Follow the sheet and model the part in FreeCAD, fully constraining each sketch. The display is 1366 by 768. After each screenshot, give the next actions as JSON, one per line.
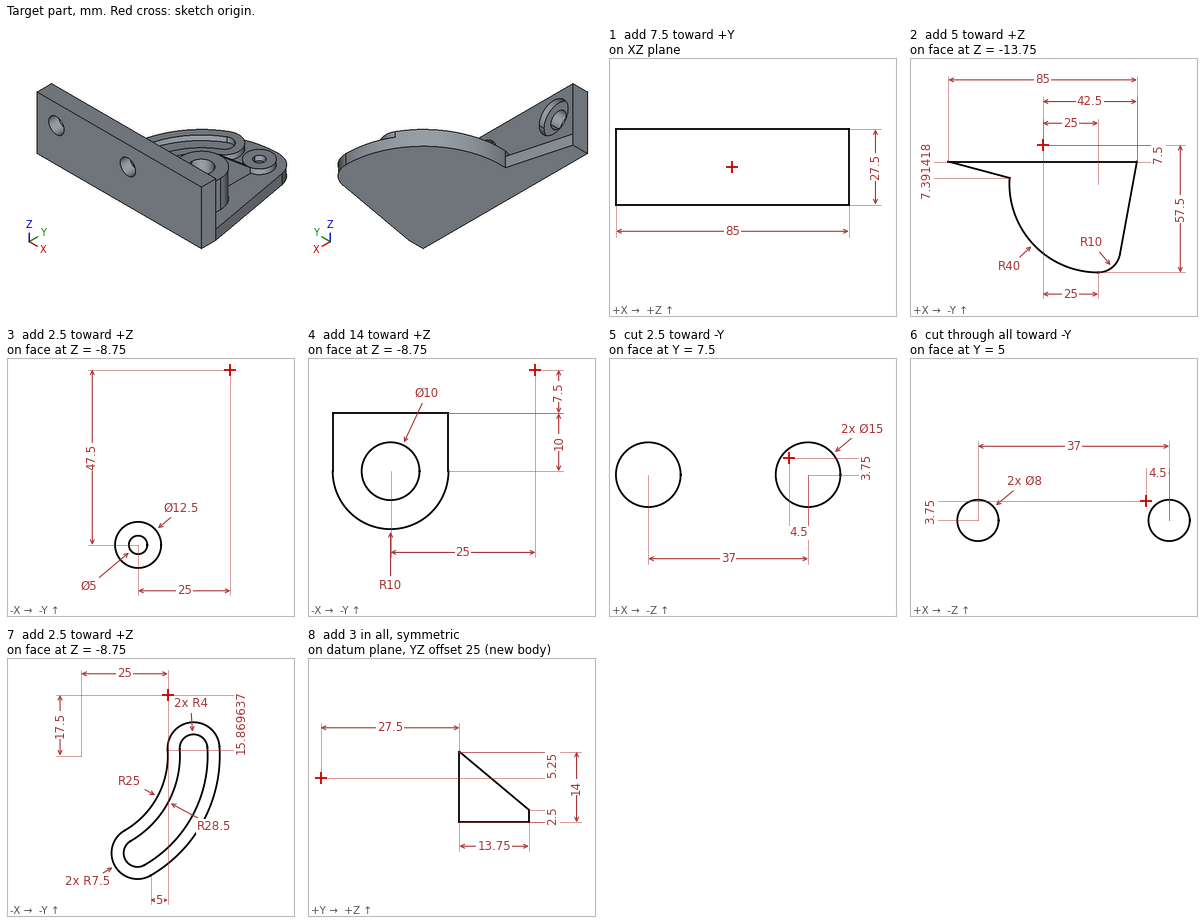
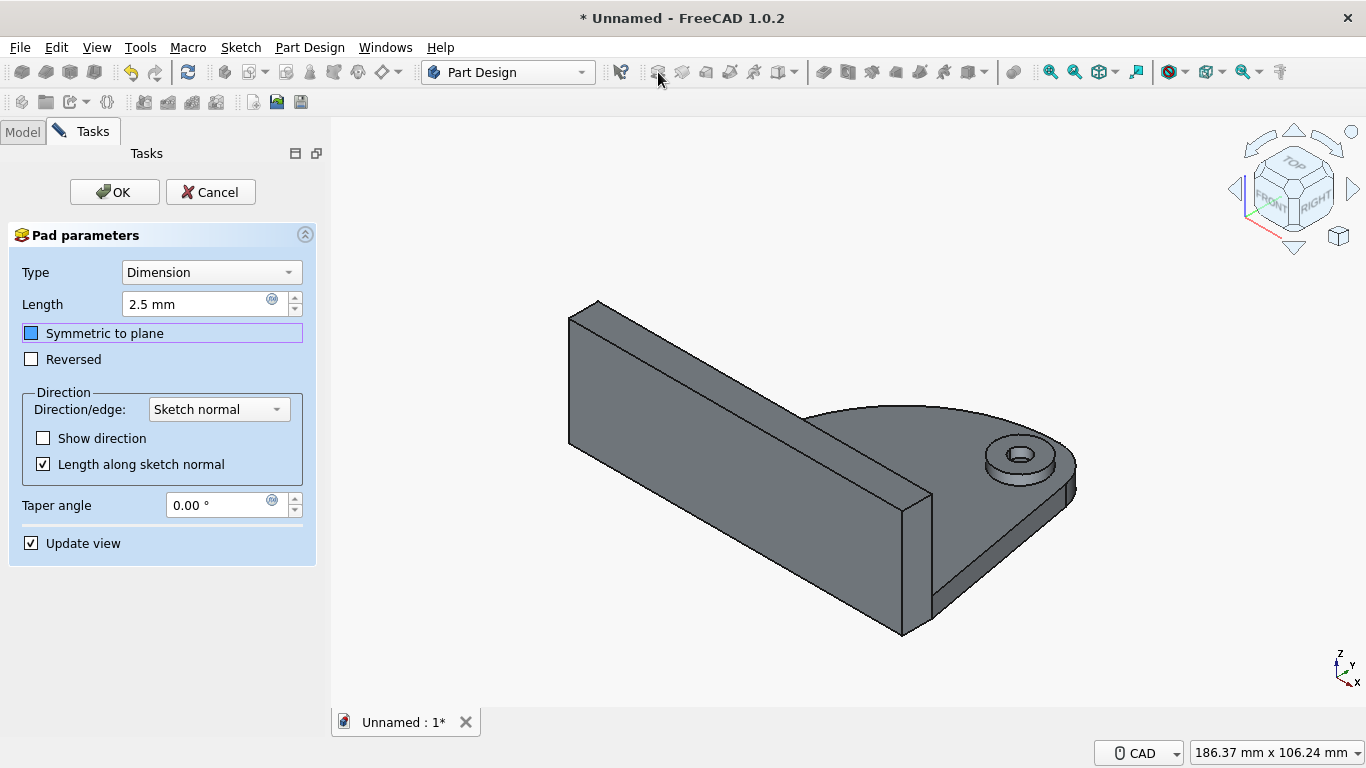
{"action": "left_click", "coordinate": [115, 192]}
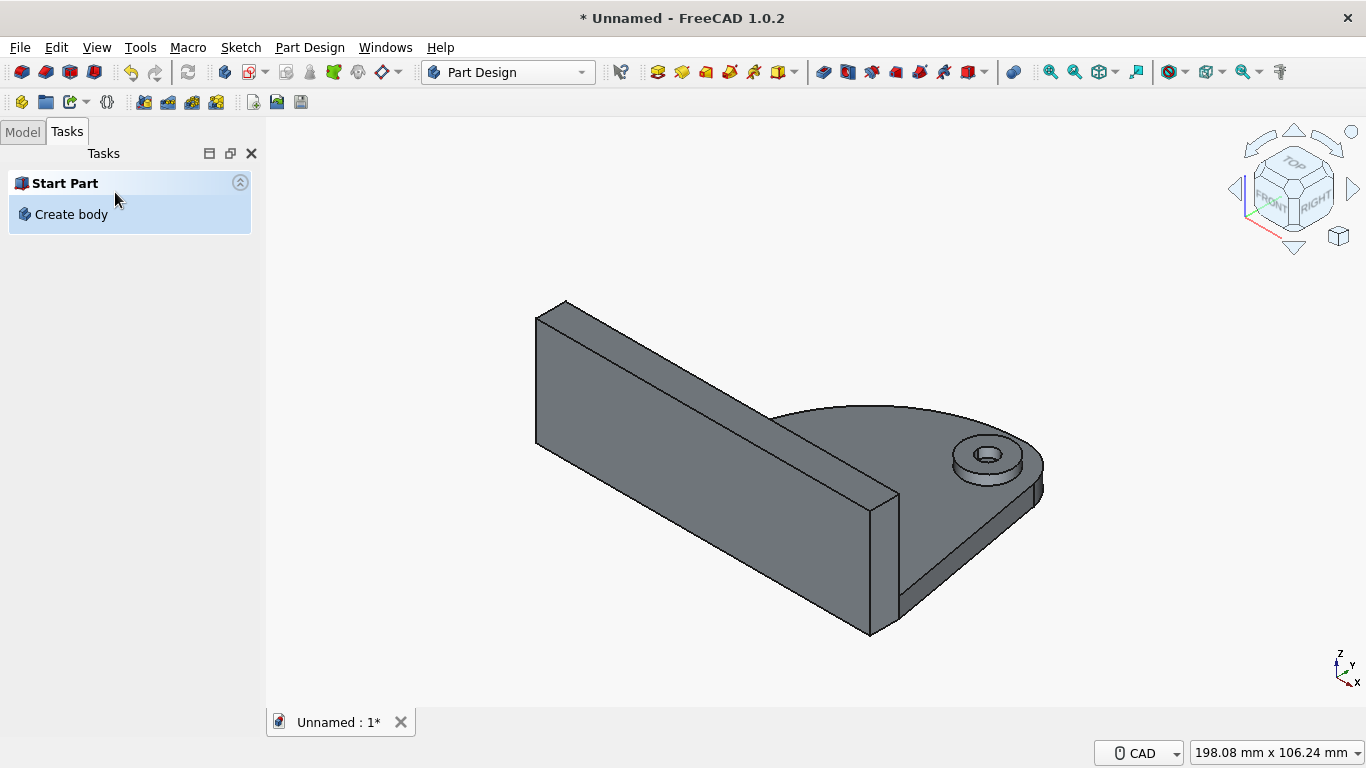
{"action": "left_click", "coordinate": [878, 470]}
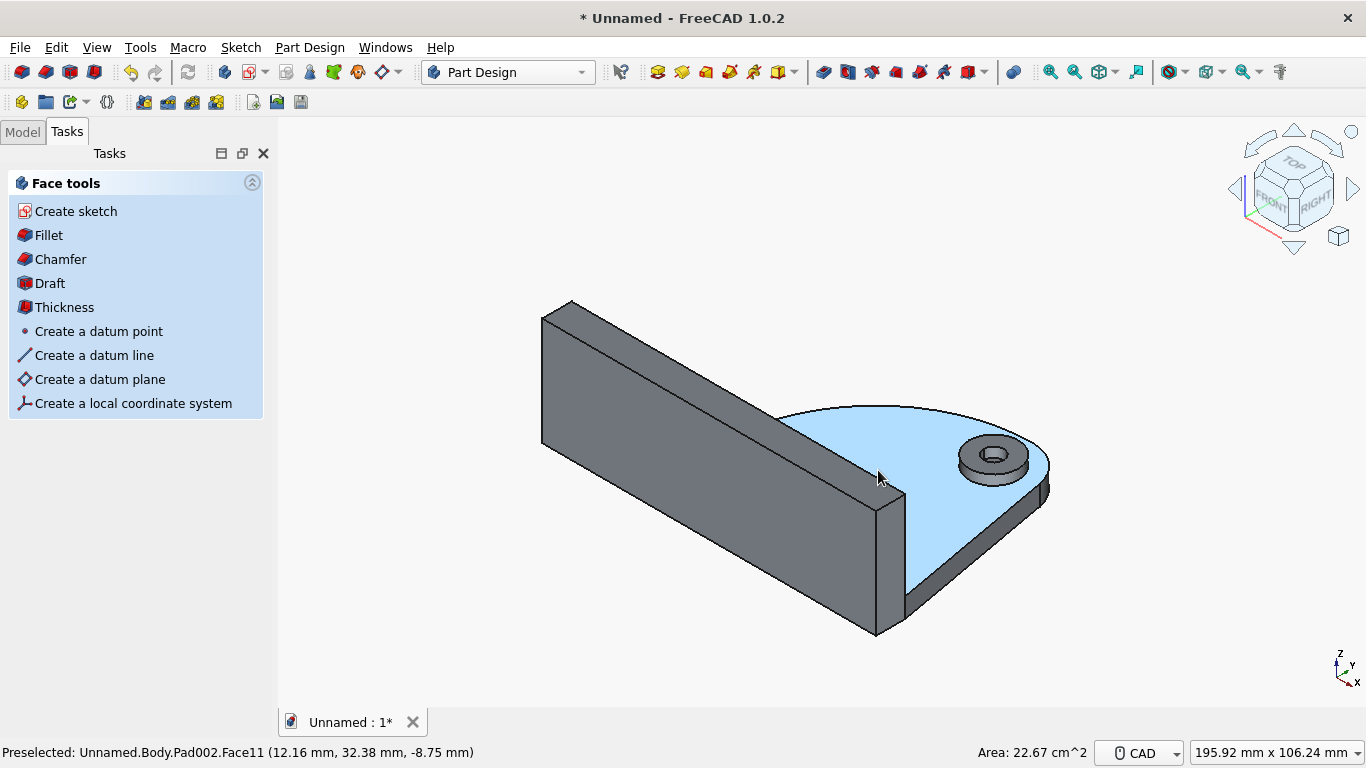
{"action": "left_click", "coordinate": [250, 72]}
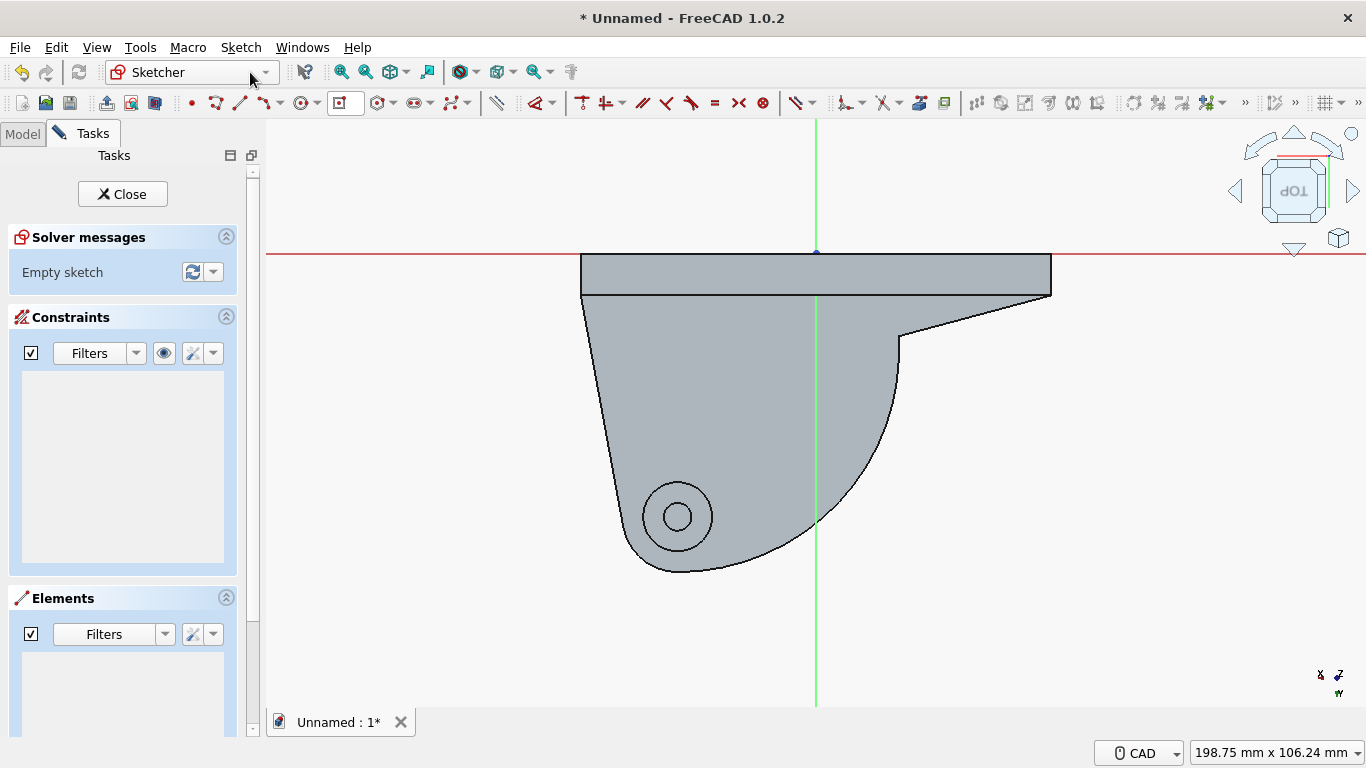
{"action": "scroll", "coordinate": [703, 282], "scroll_direction": "up", "scroll_amount": 5}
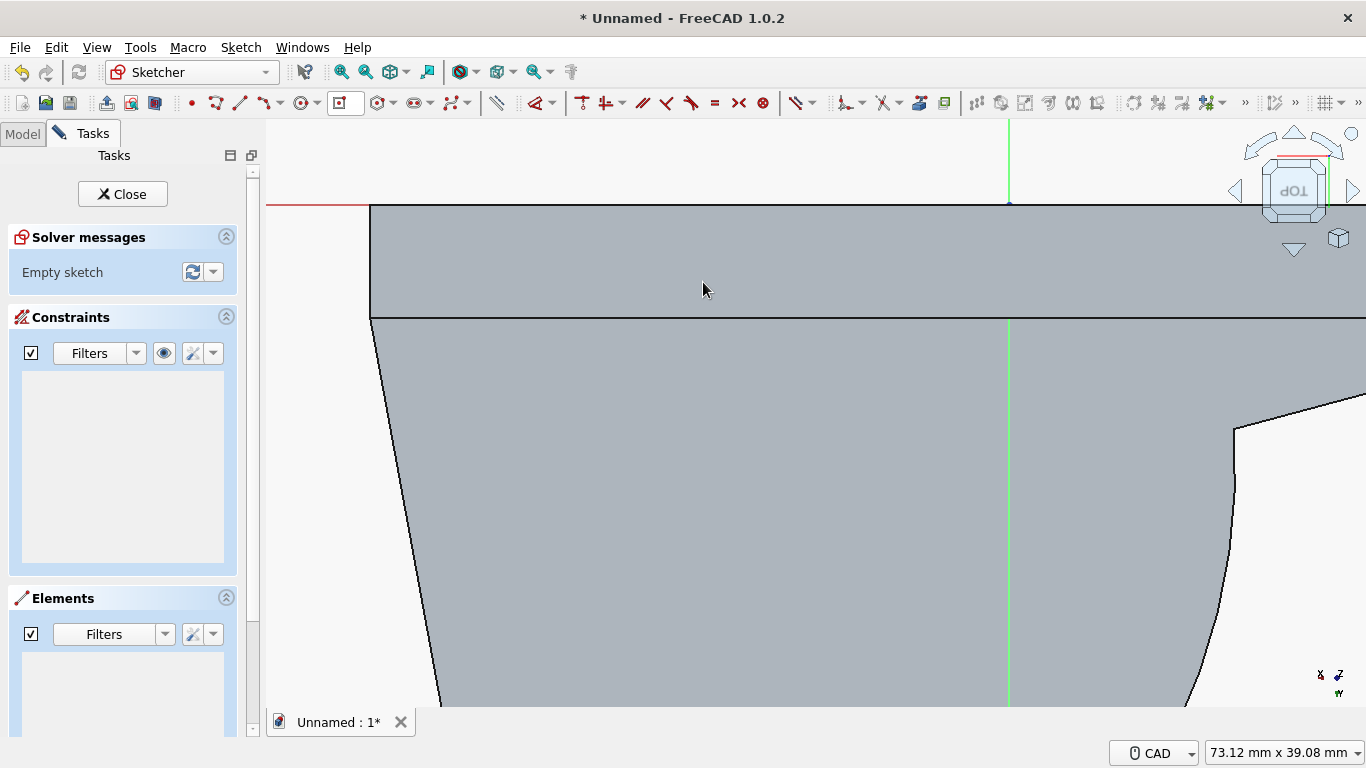
{"action": "left_click", "coordinate": [216, 104]}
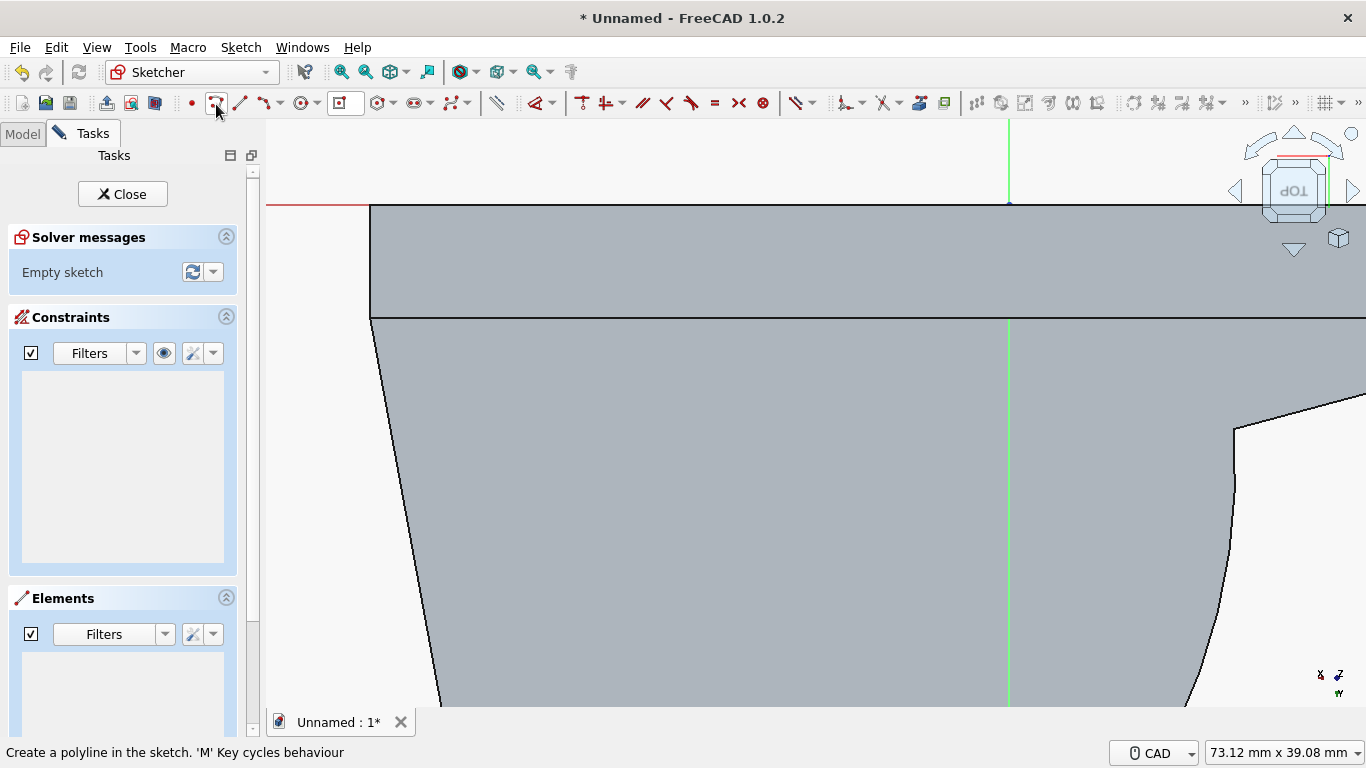
{"action": "left_click", "coordinate": [784, 468]}
{"action": "left_click", "coordinate": [784, 318]}
{"action": "left_click", "coordinate": [483, 318]}
{"action": "left_click", "coordinate": [483, 468]}
{"action": "right_click", "coordinate": [483, 468]}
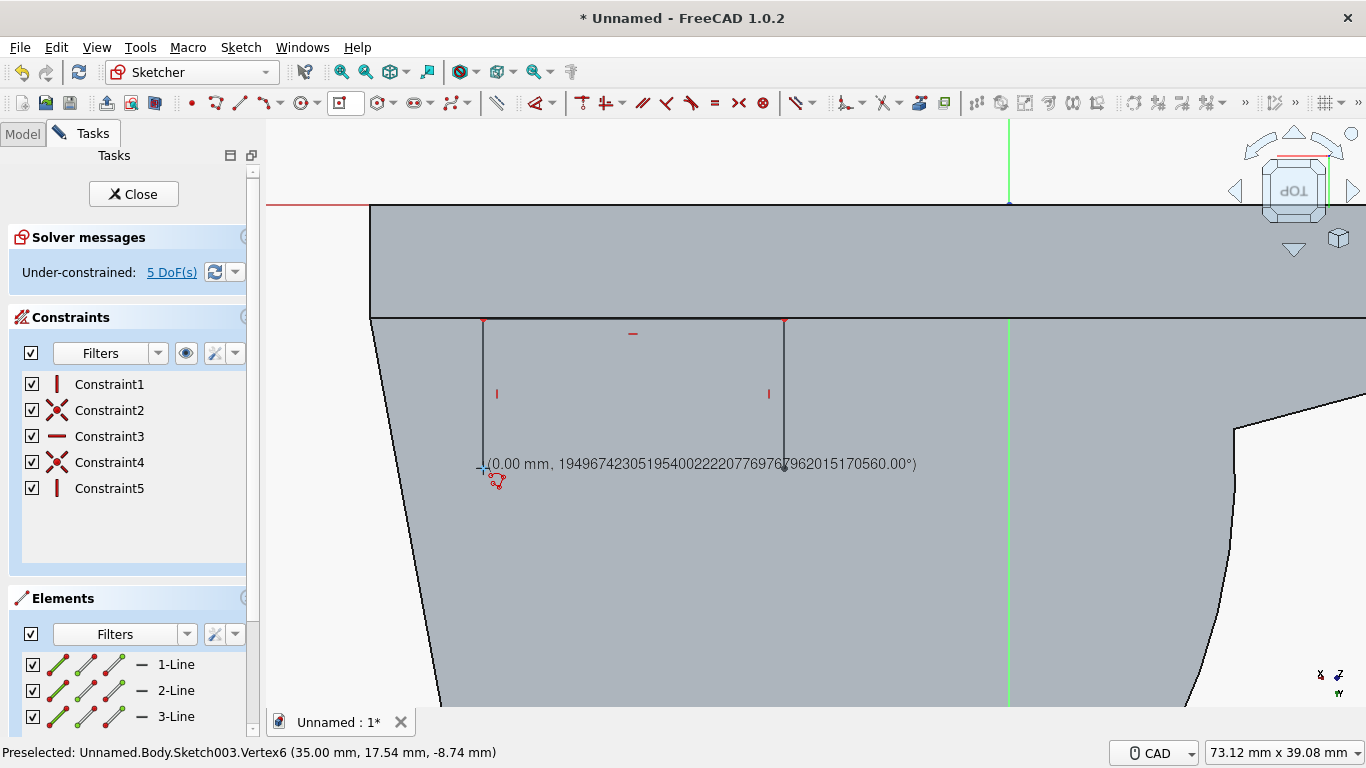
{"action": "left_click", "coordinate": [264, 104]}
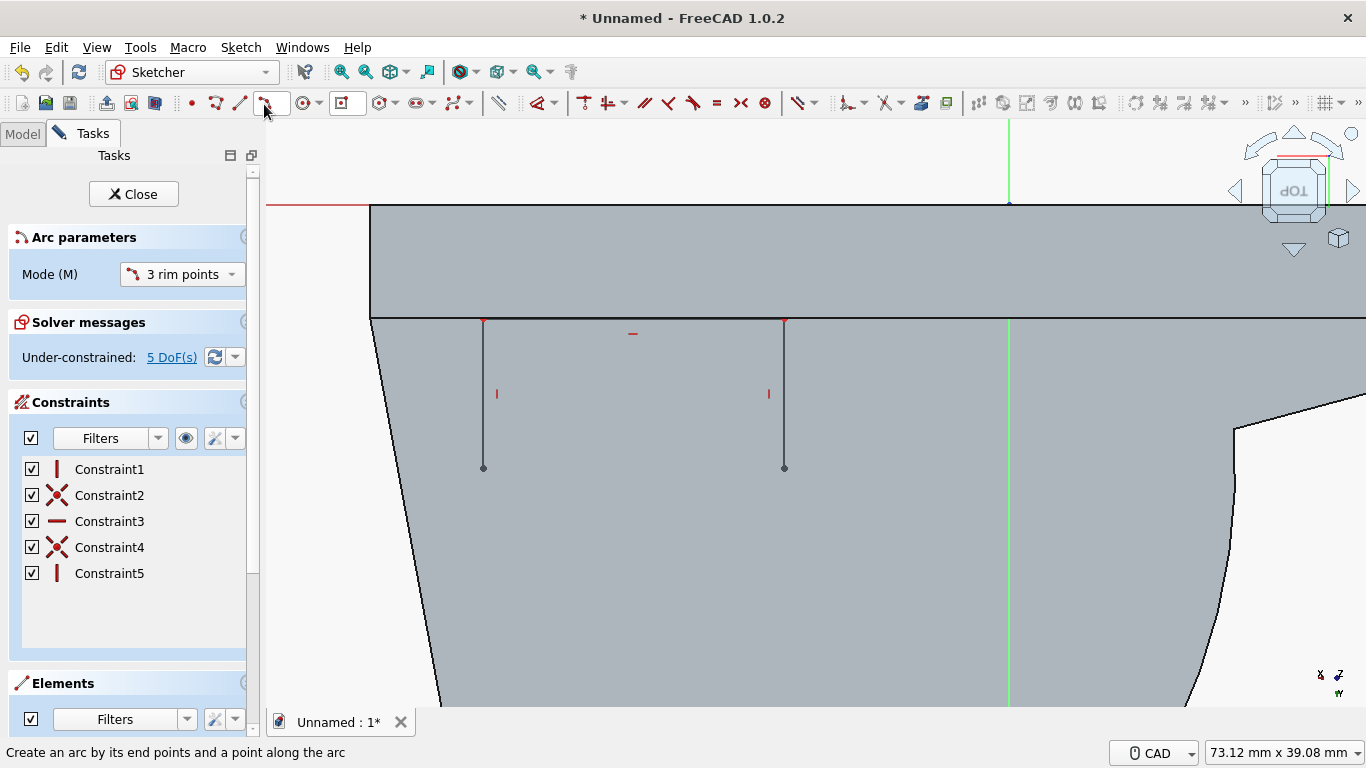
{"action": "left_click", "coordinate": [483, 469]}
{"action": "left_click", "coordinate": [784, 469]}
{"action": "left_click", "coordinate": [633, 619]}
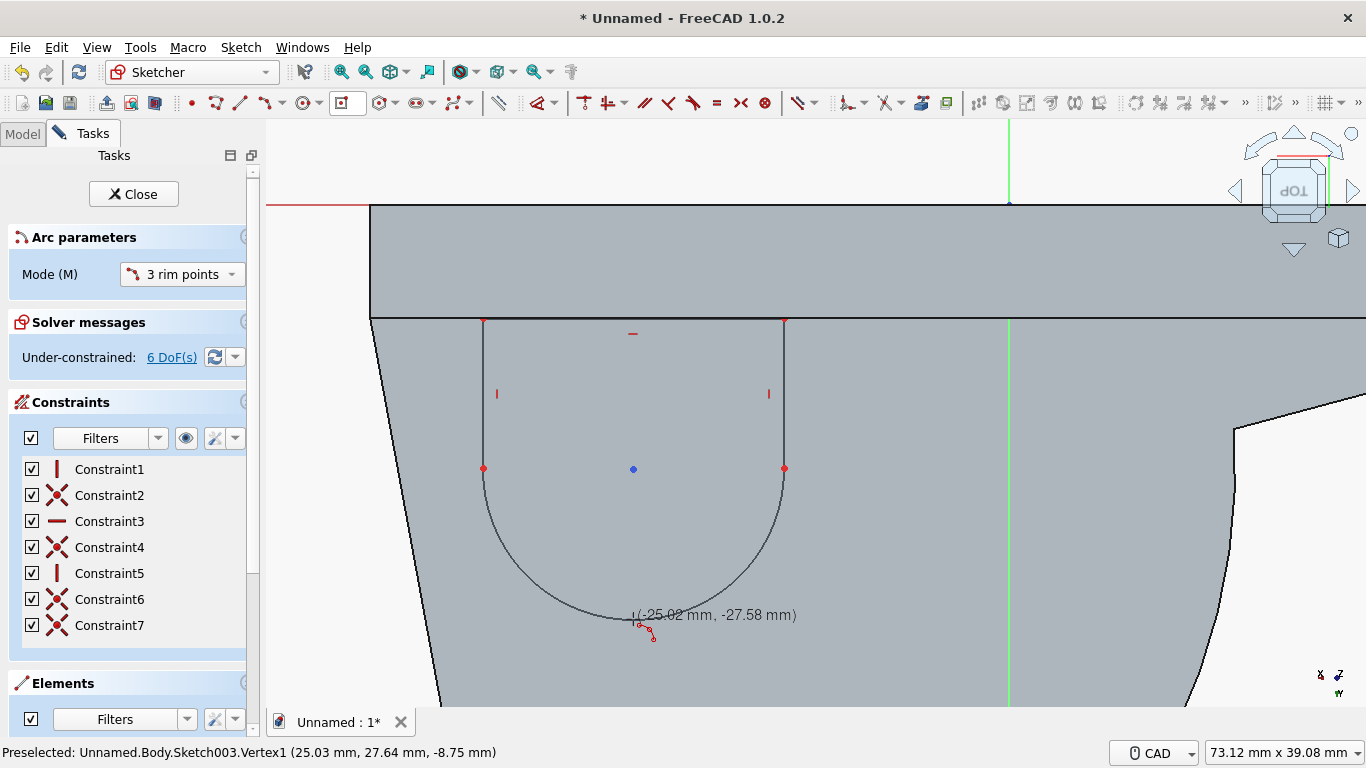
{"action": "left_click", "coordinate": [304, 104]}